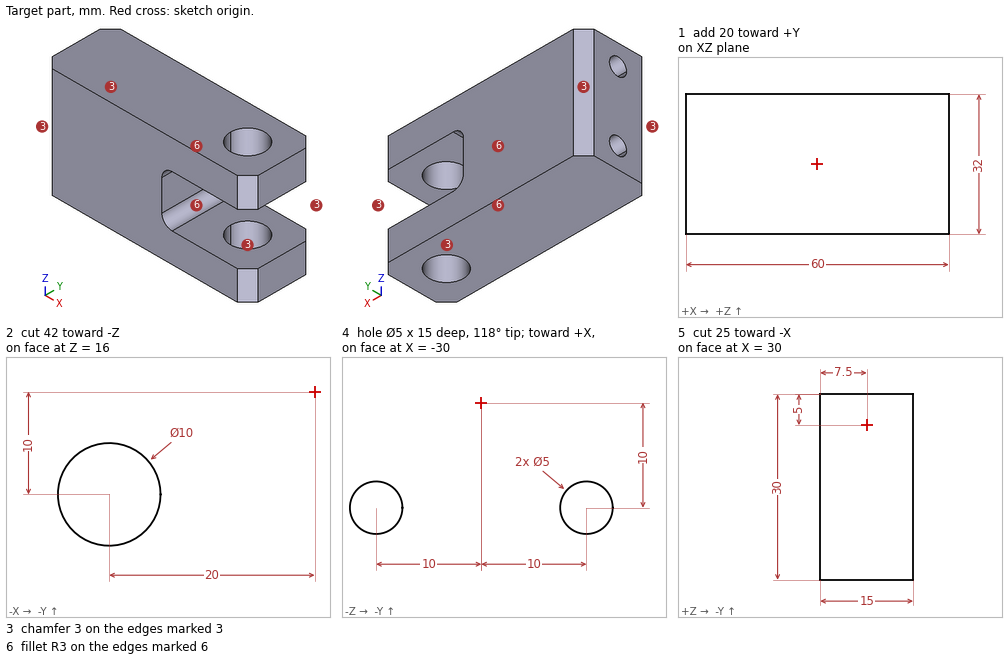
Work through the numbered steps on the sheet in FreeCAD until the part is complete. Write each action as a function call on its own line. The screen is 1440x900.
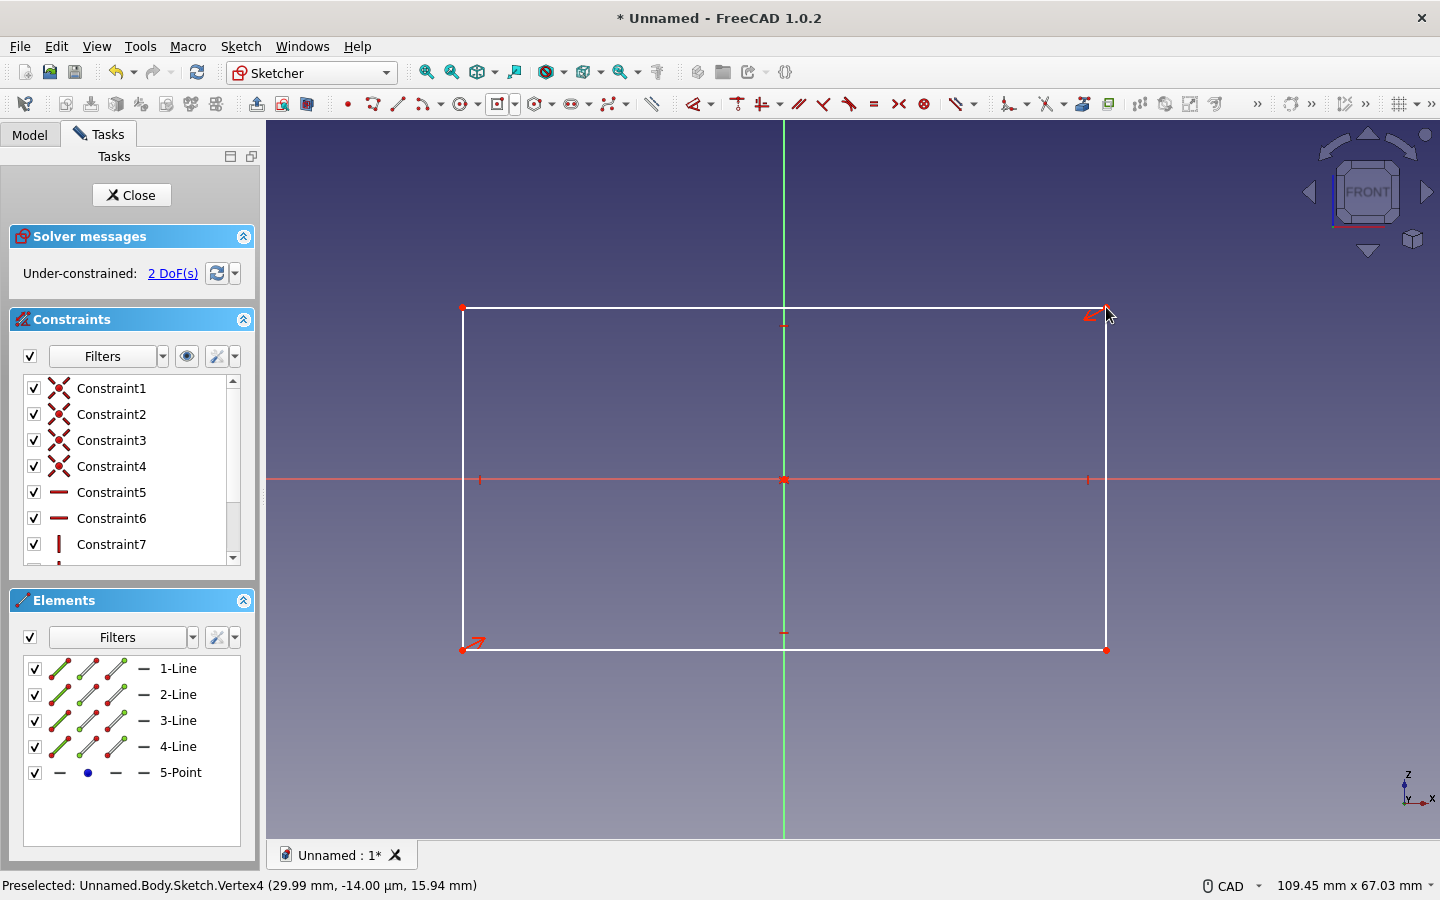
click(656, 650)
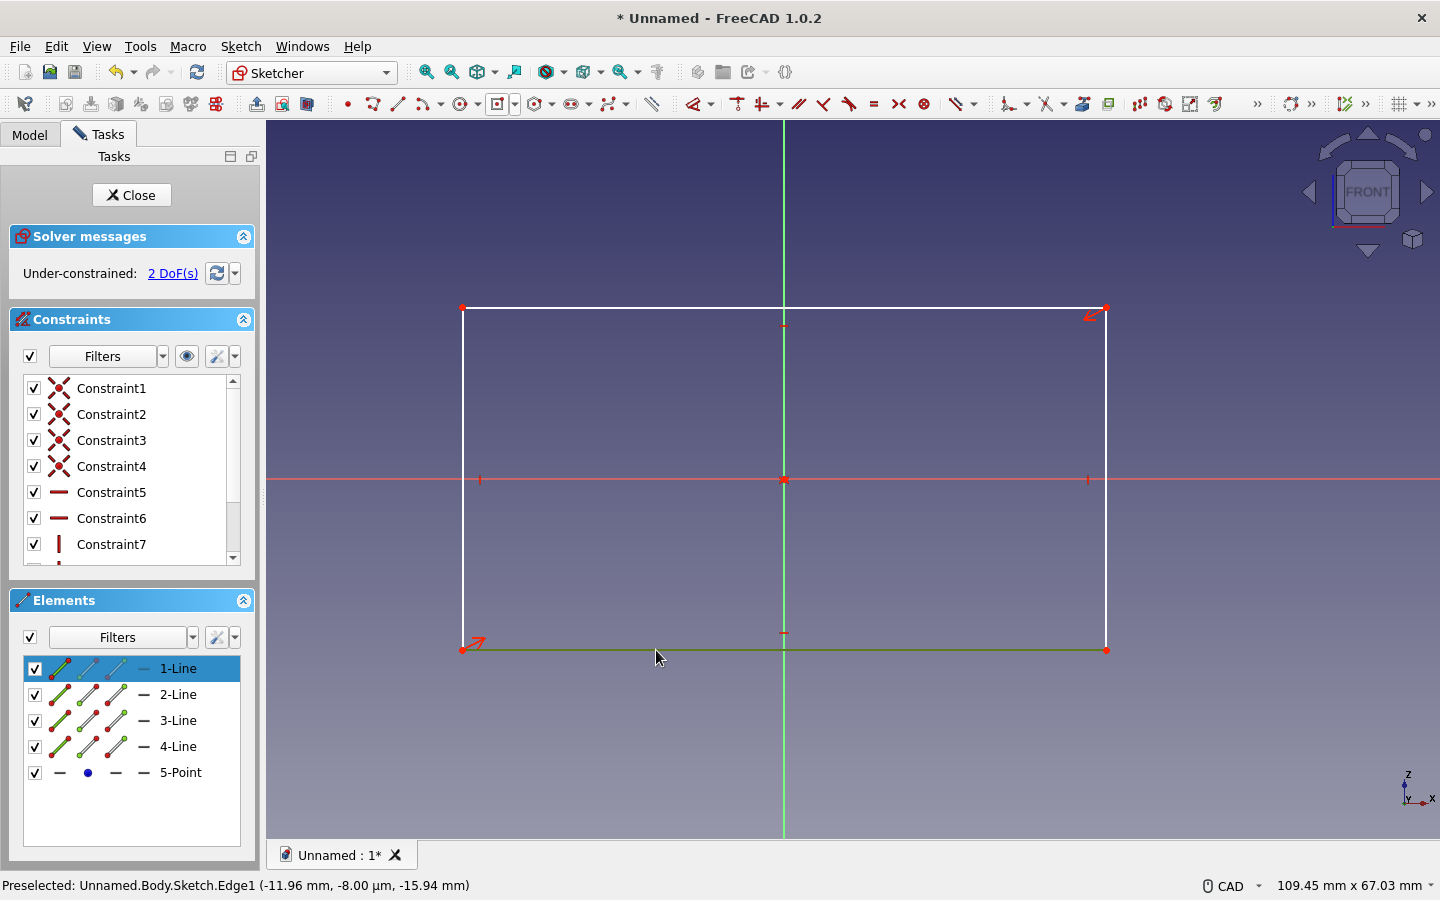
click(710, 104)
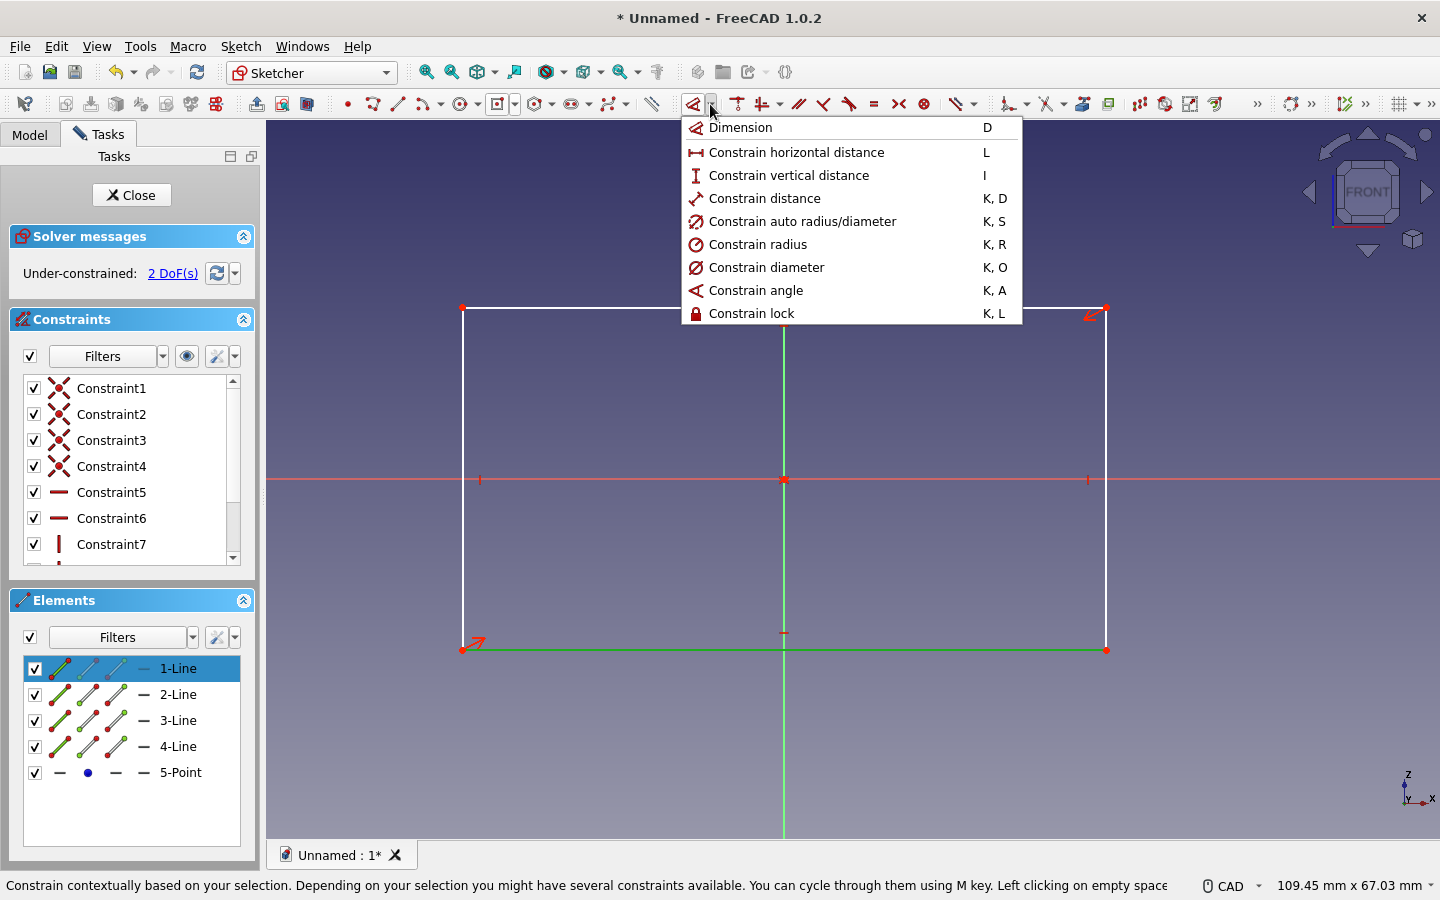
click(852, 152)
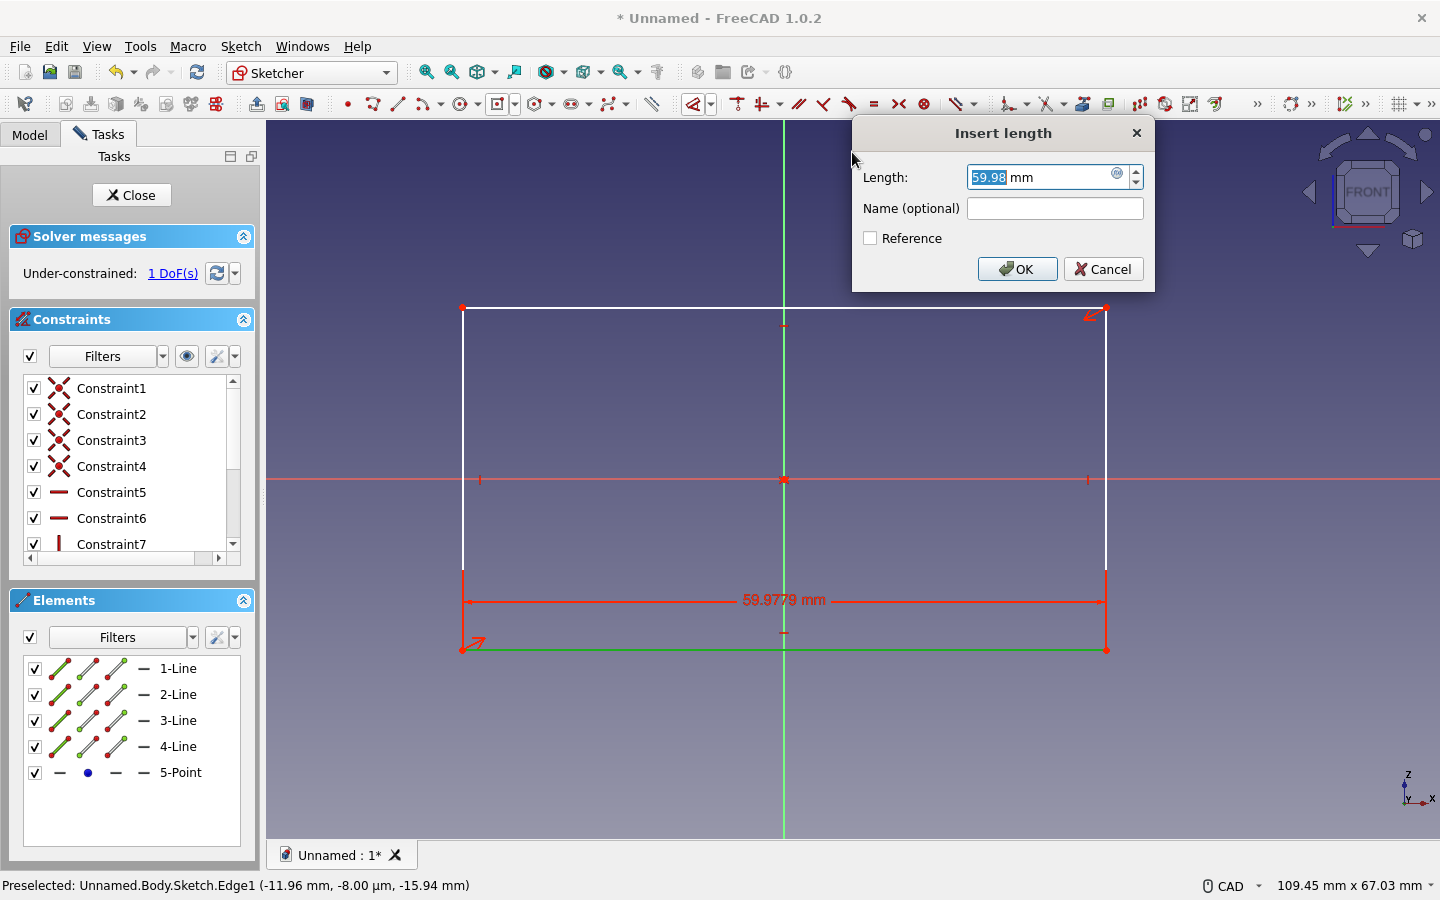
text(60)
key(Return)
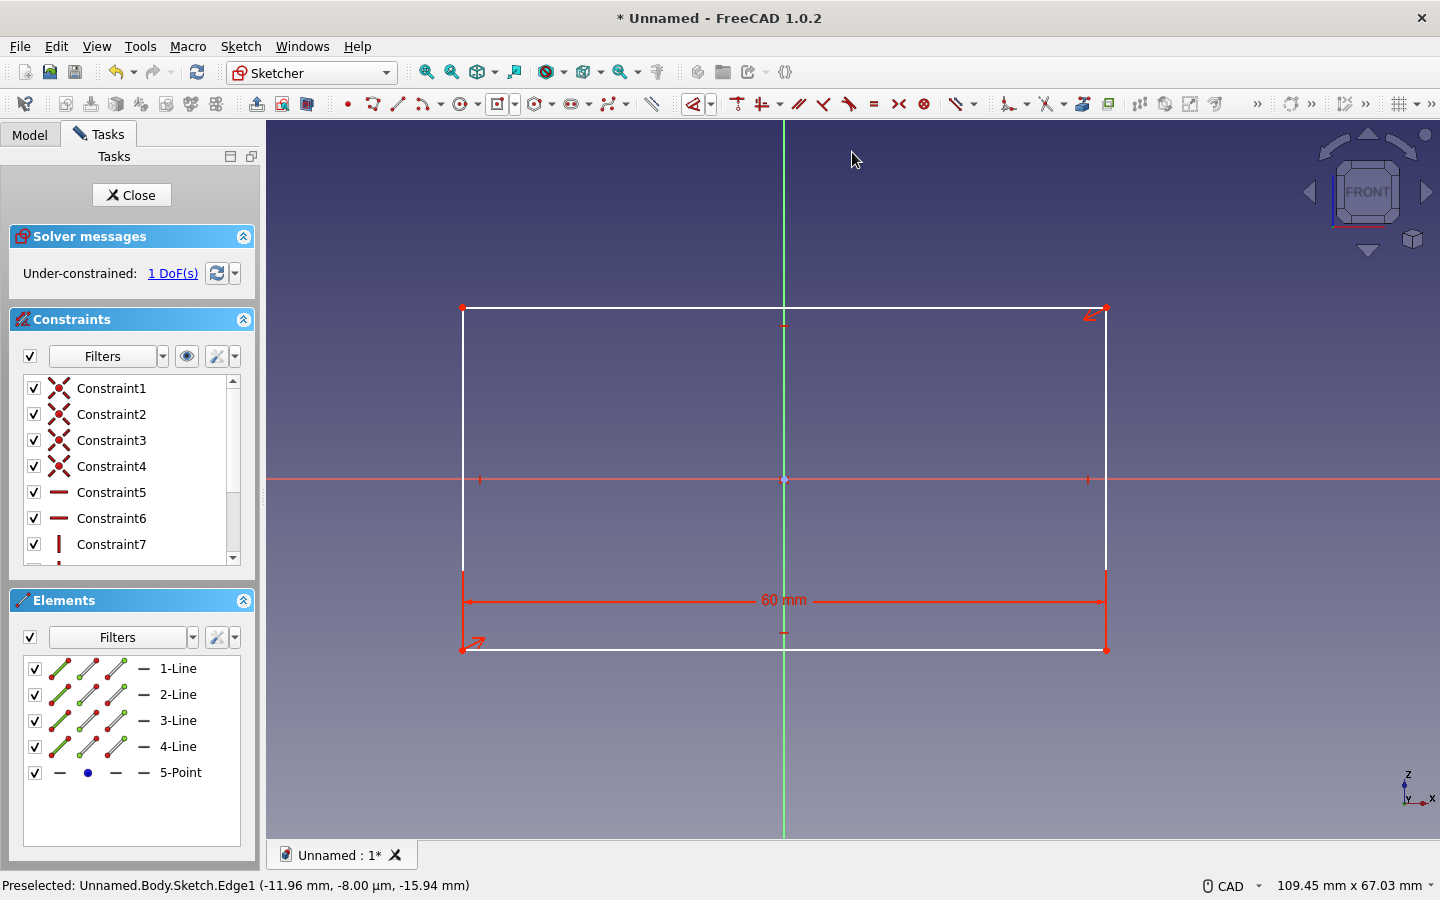
click(1106, 547)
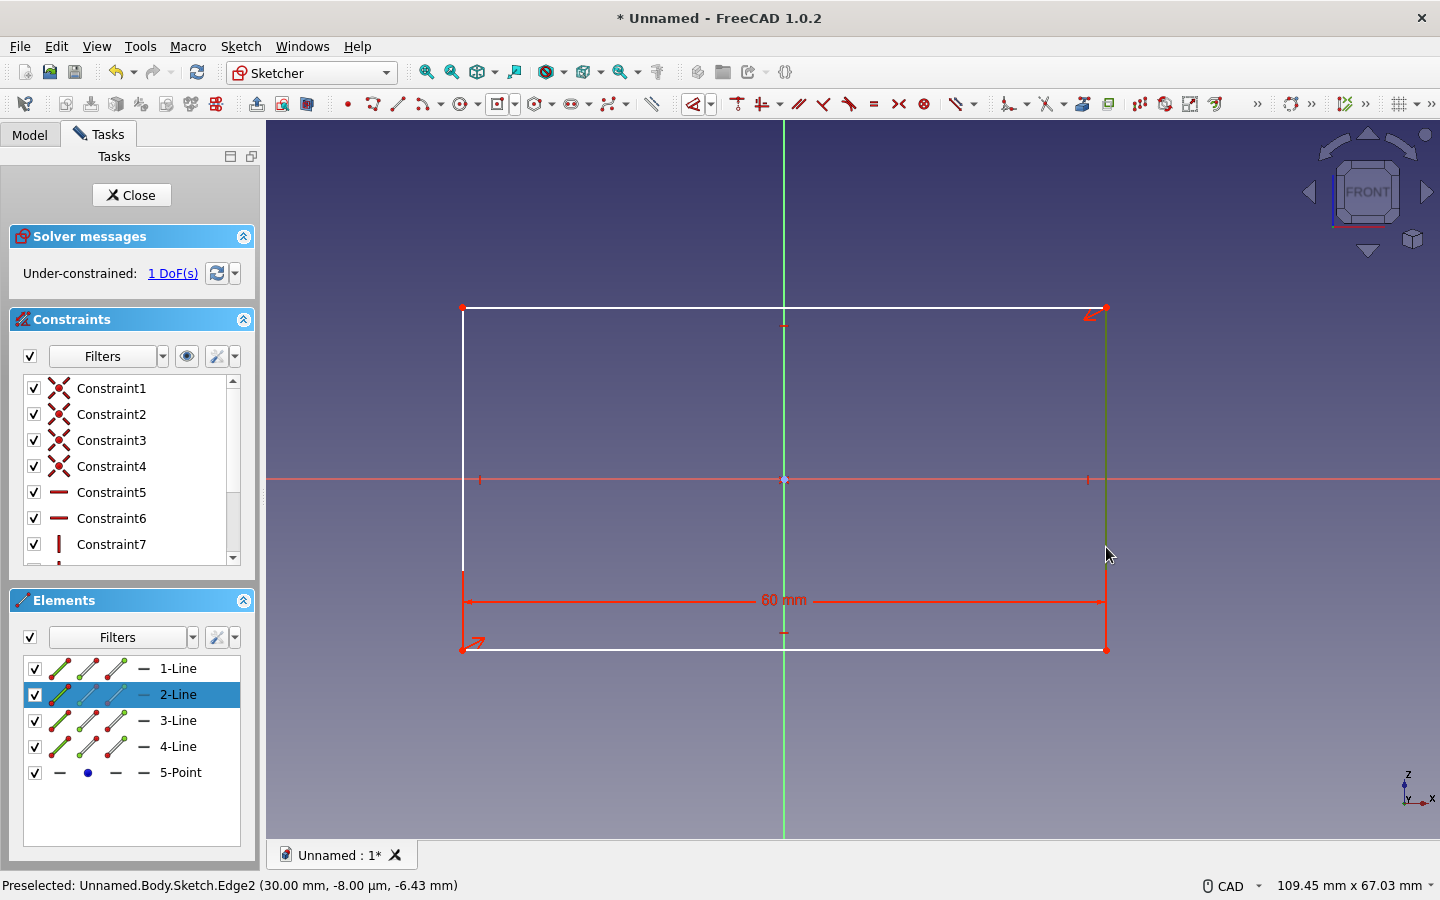
key(i)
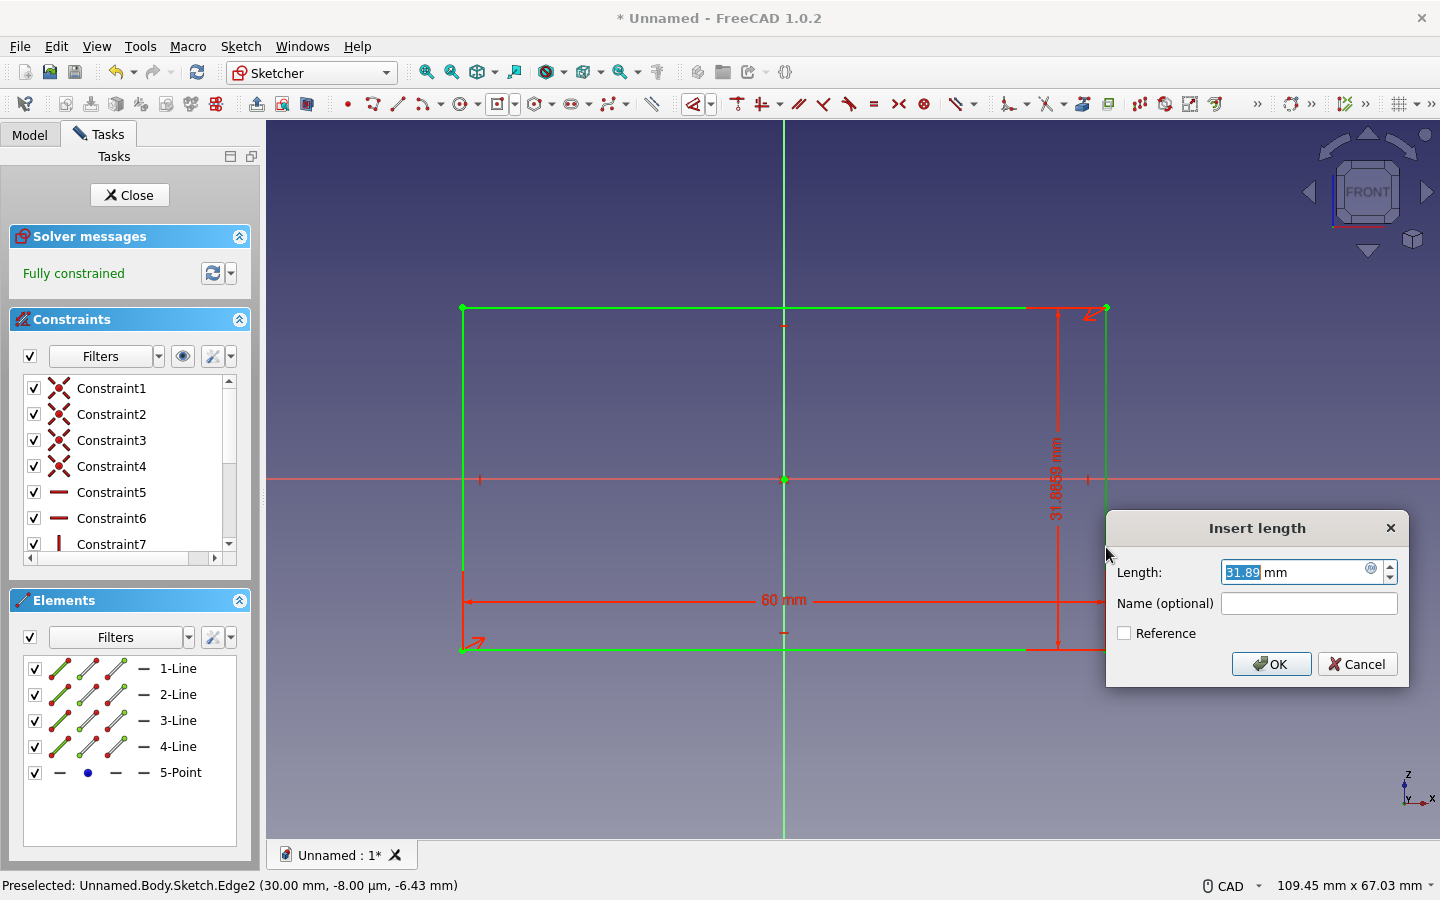
text(32)
key(Return)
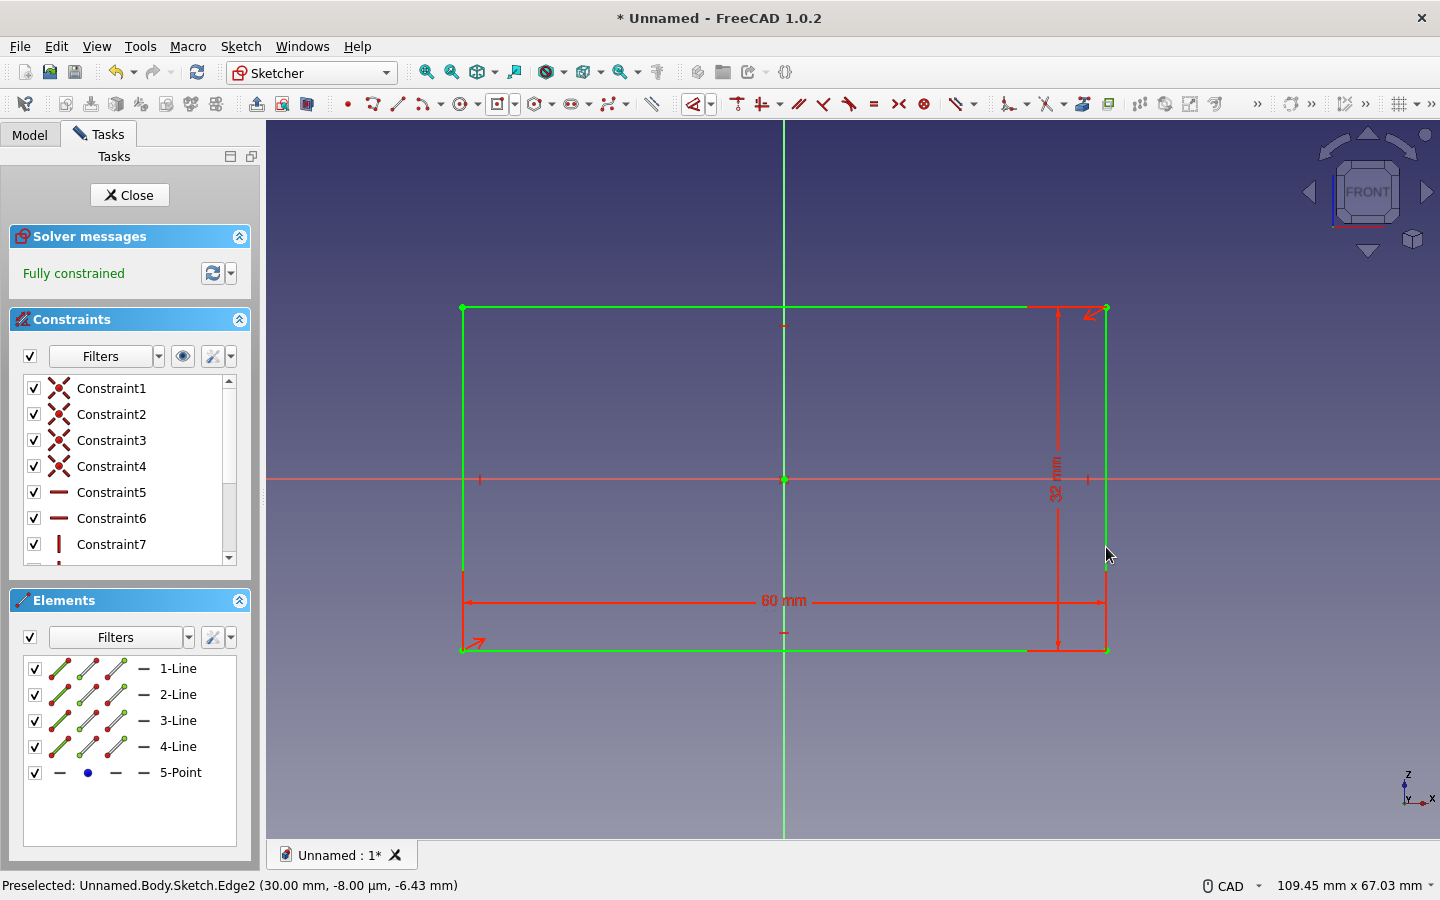
click(130, 195)